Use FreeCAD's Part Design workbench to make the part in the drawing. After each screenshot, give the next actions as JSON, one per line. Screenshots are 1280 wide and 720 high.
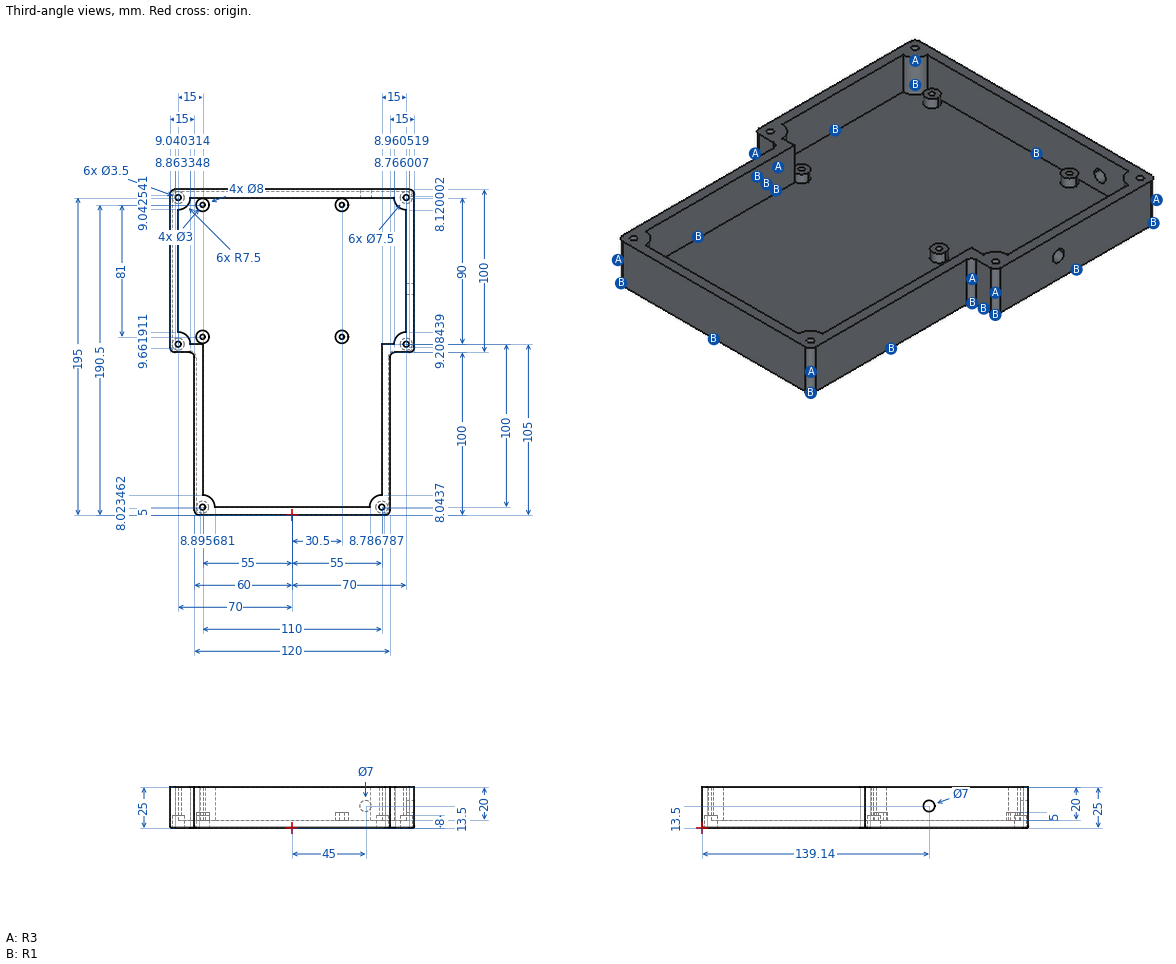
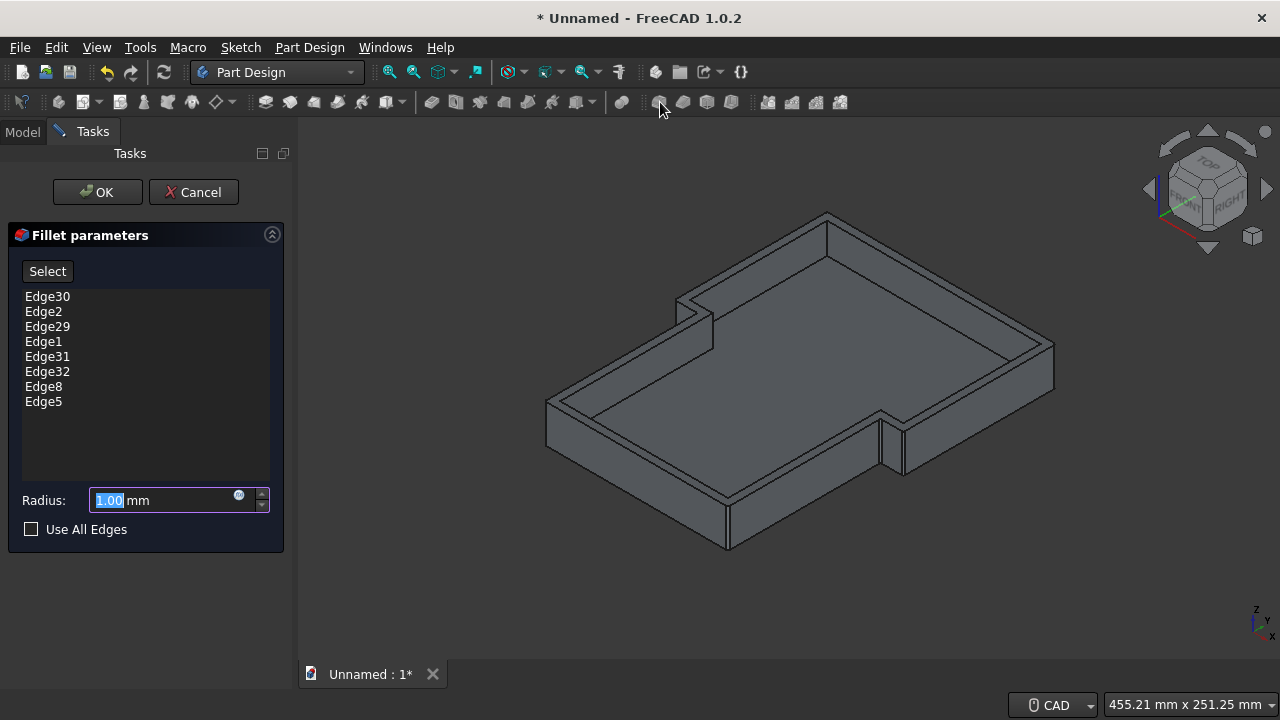
{"action": "type", "text": "3"}
{"action": "key", "text": "Tab"}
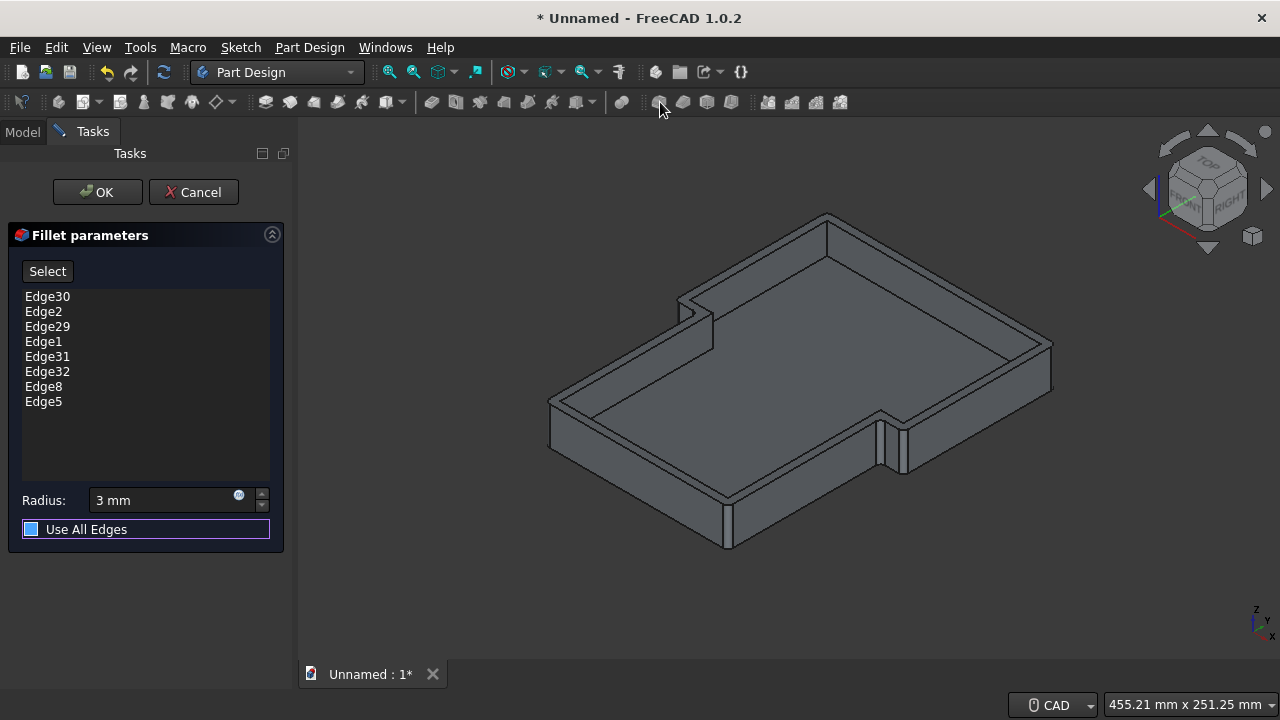
{"action": "left_click", "coordinate": [98, 192]}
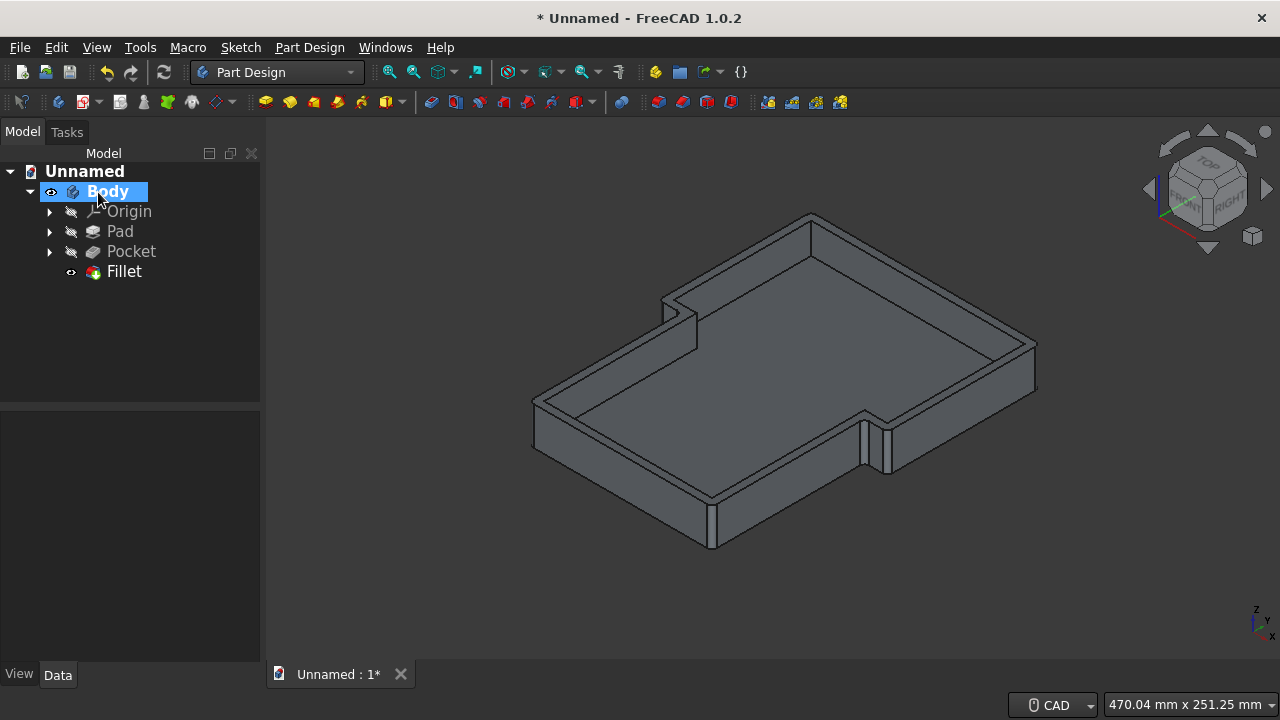
{"action": "key", "text": "2"}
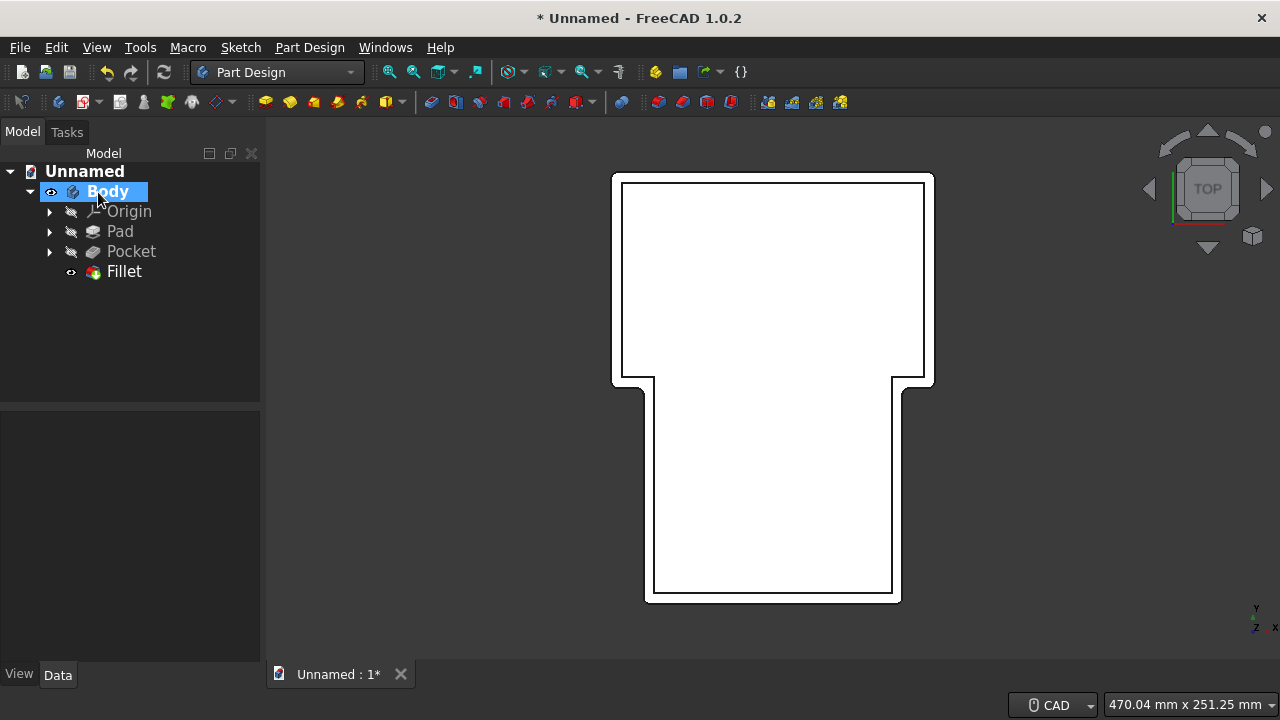
{"action": "key", "text": "0"}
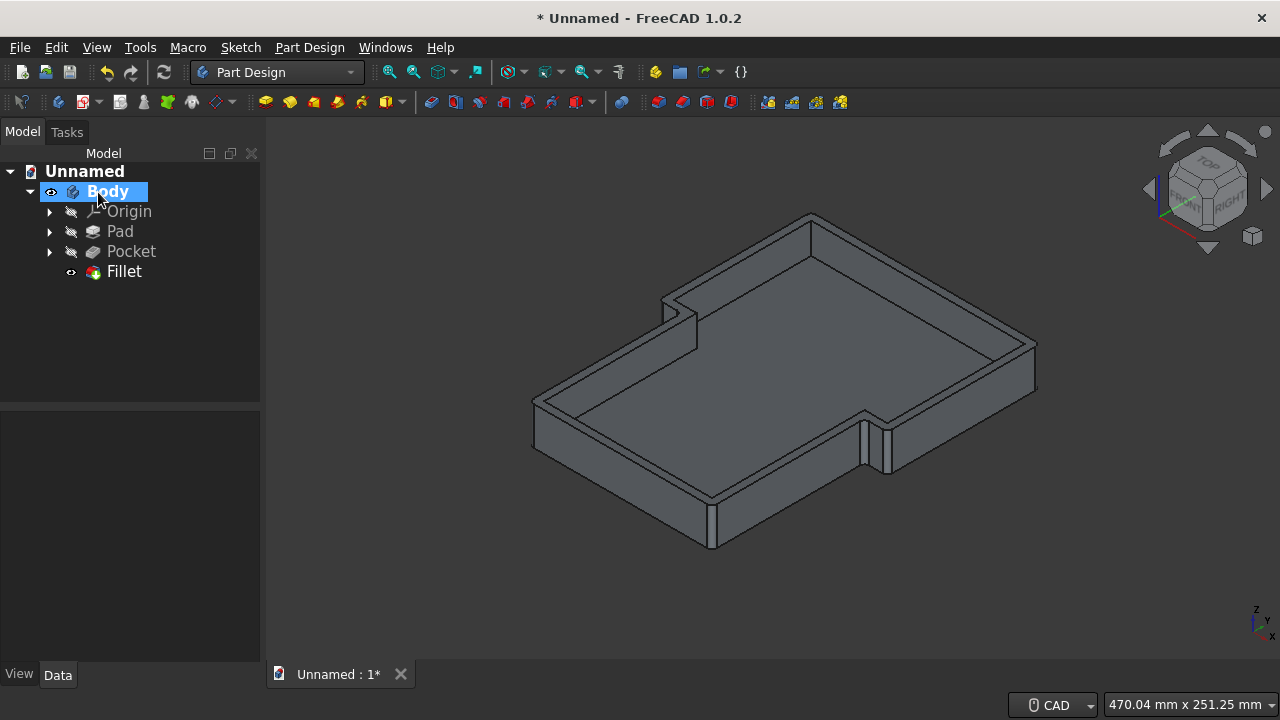
{"action": "key", "text": "1"}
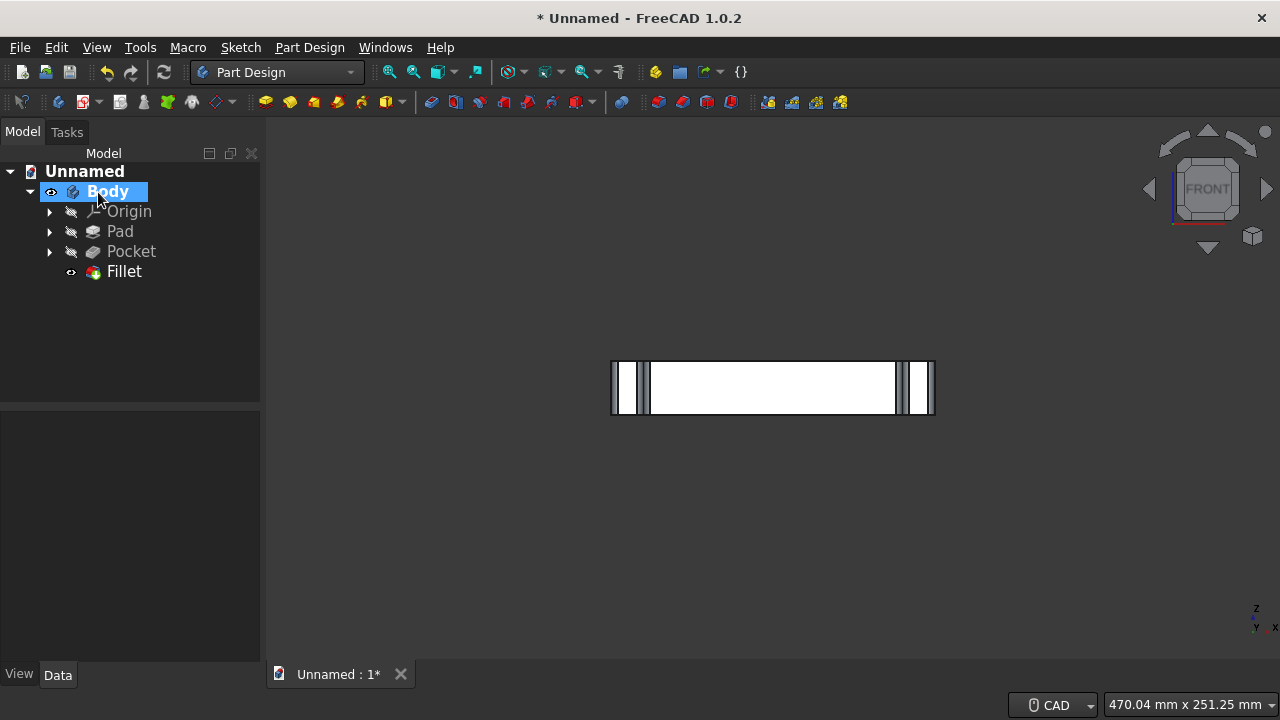
{"action": "left_click", "coordinate": [390, 72]}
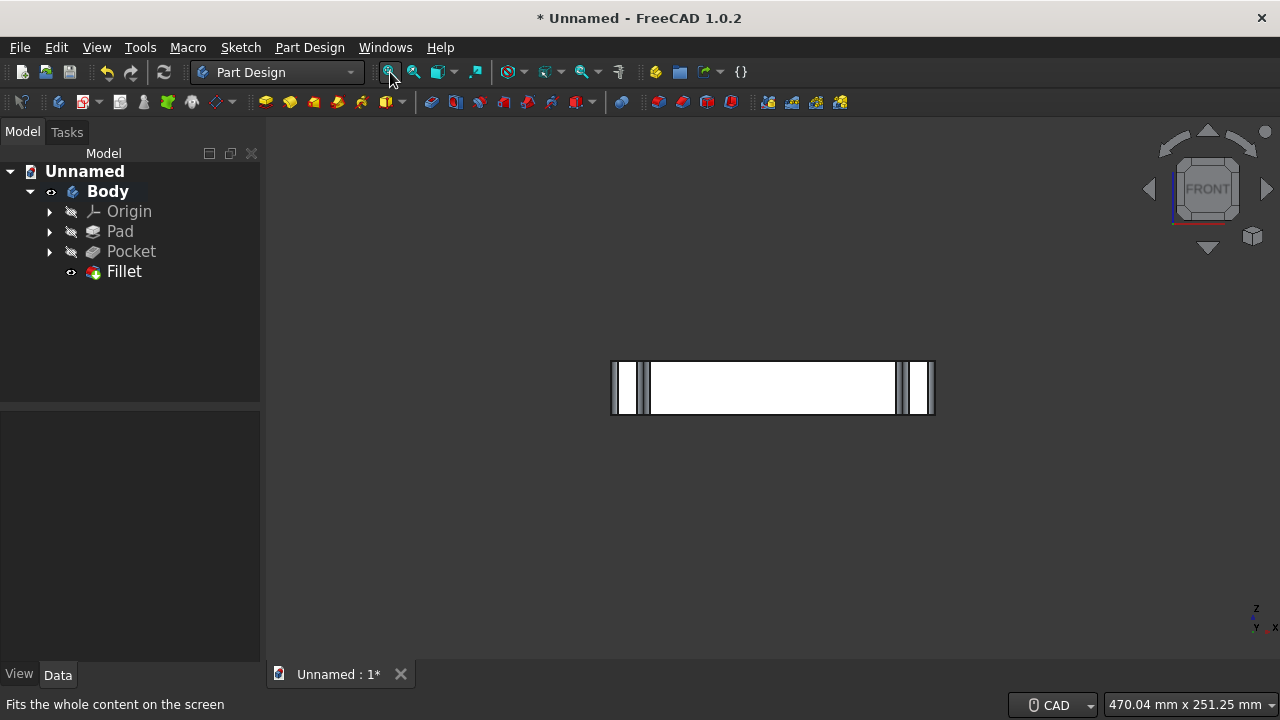
{"action": "key", "text": "3"}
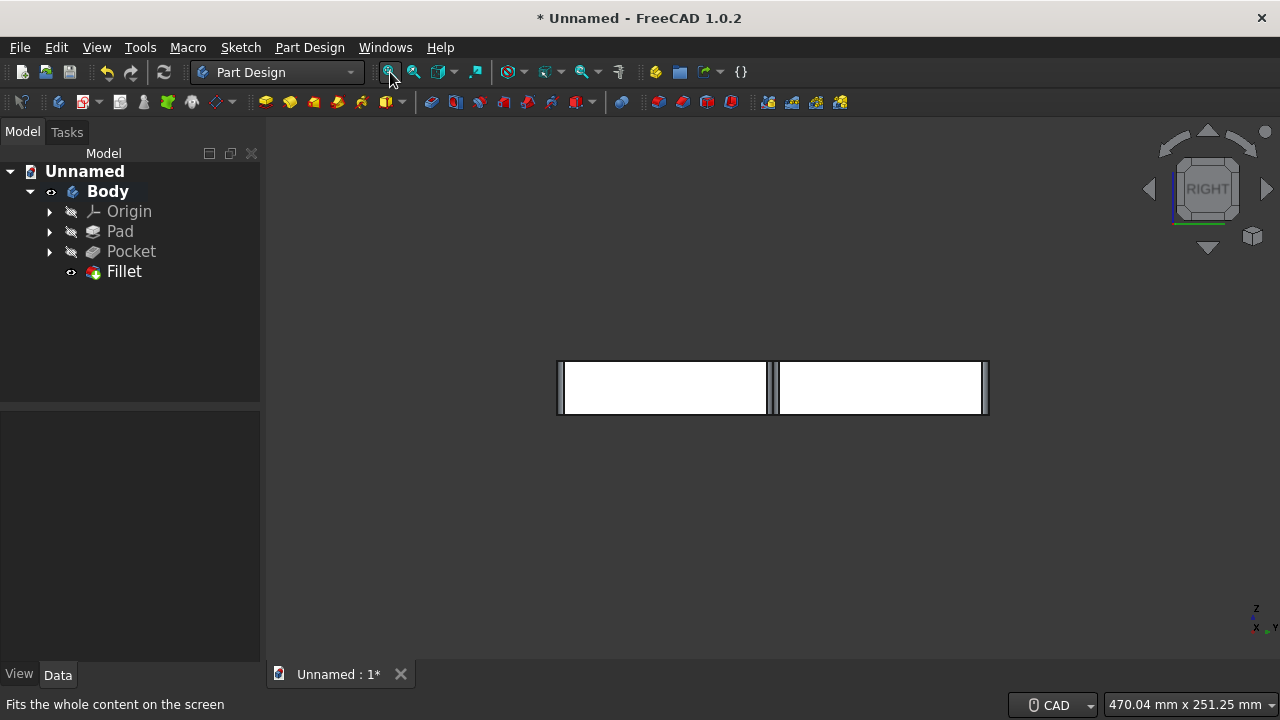
{"action": "key", "text": "v f"}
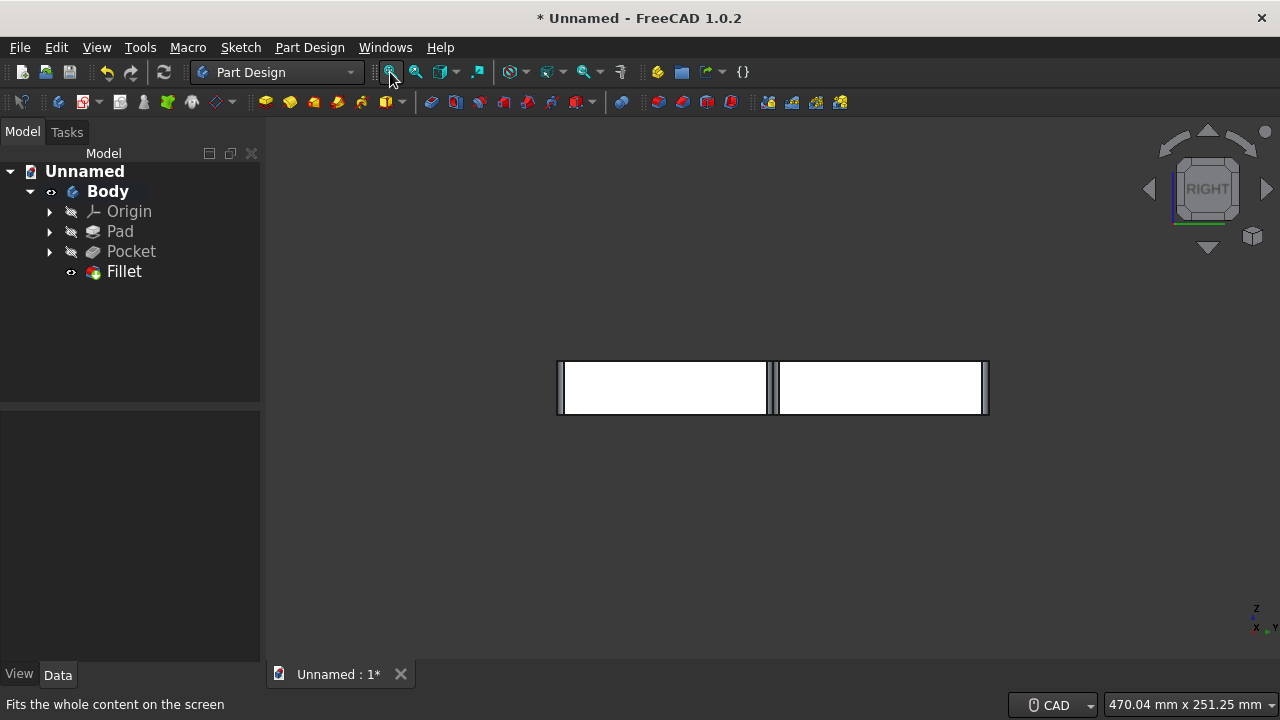
{"action": "key", "text": "5"}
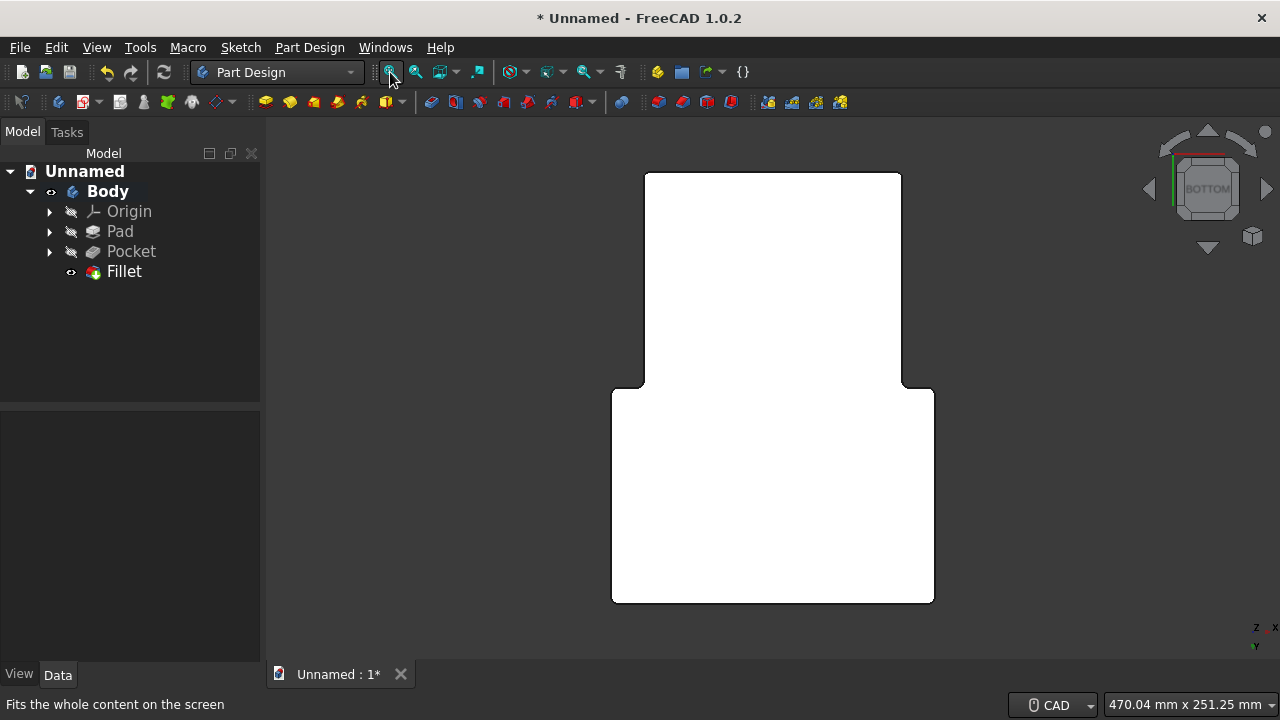
{"action": "left_click", "coordinate": [773, 449]}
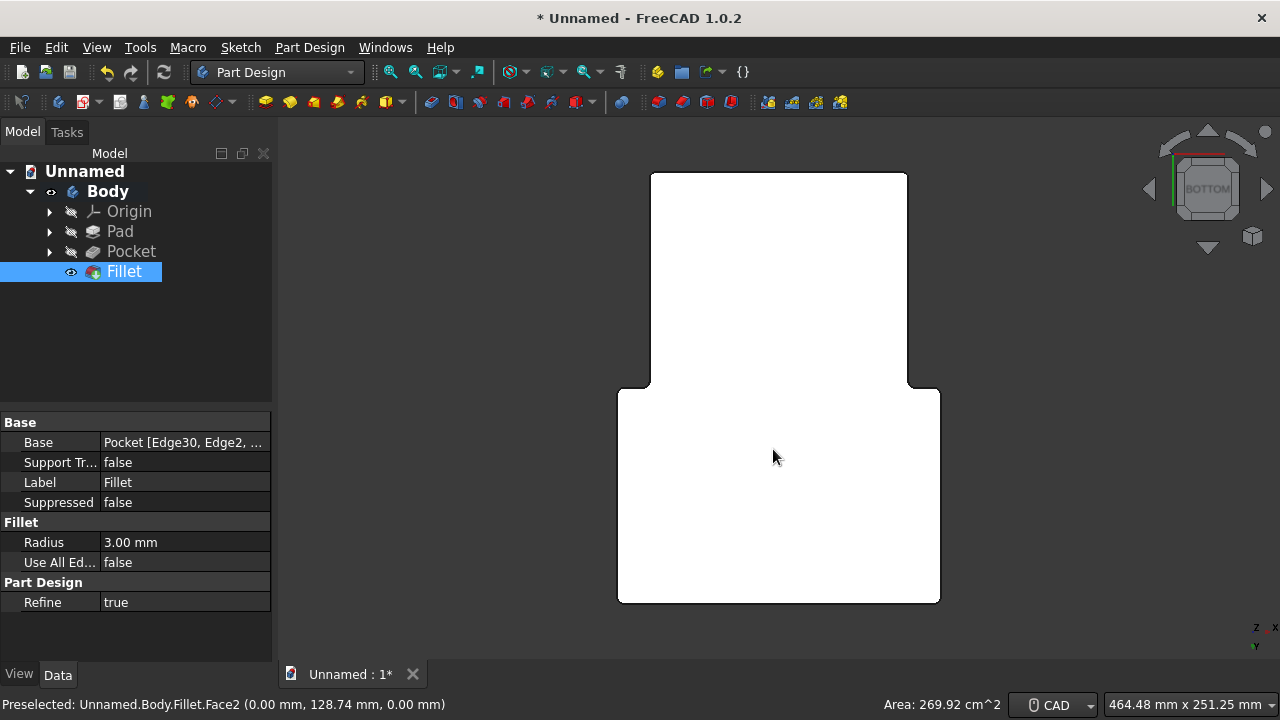
{"action": "left_click", "coordinate": [660, 102]}